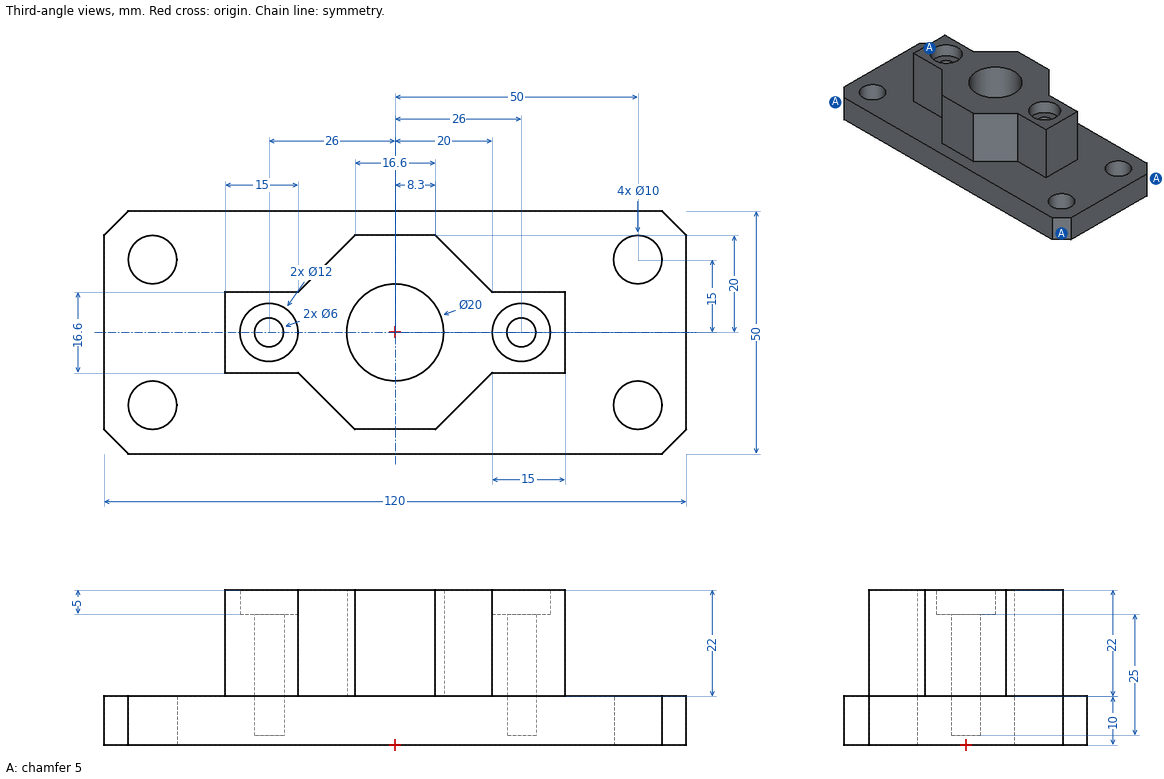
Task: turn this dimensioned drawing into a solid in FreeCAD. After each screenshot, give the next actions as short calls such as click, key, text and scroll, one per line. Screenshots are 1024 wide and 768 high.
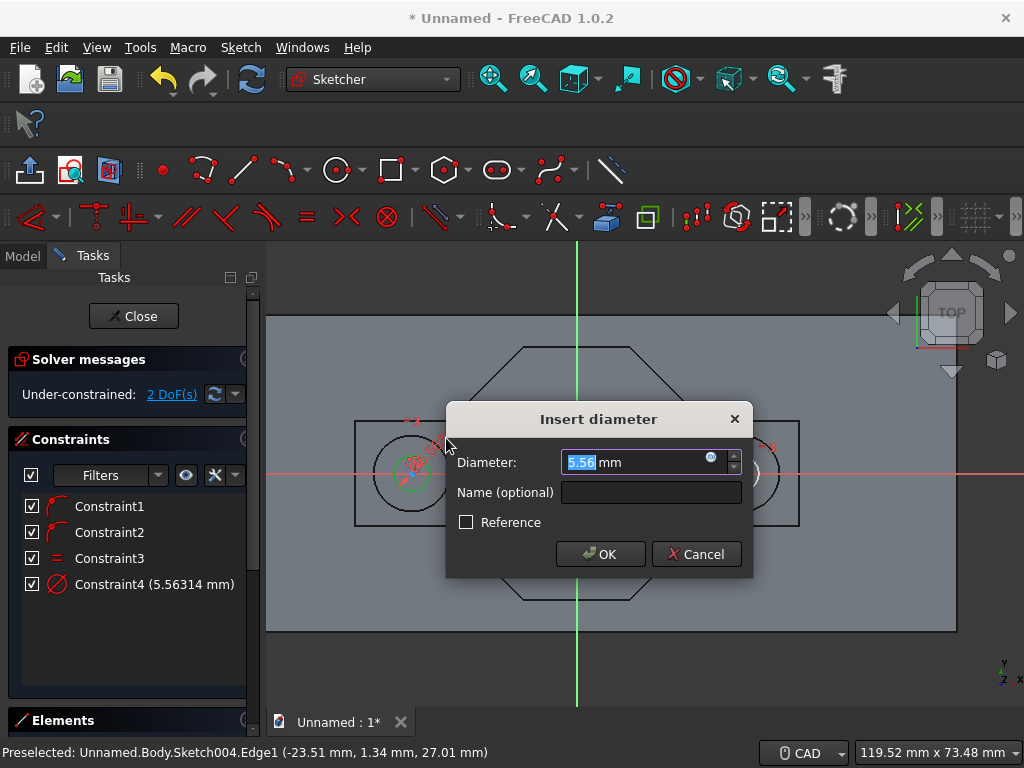
text(6)
key(Return)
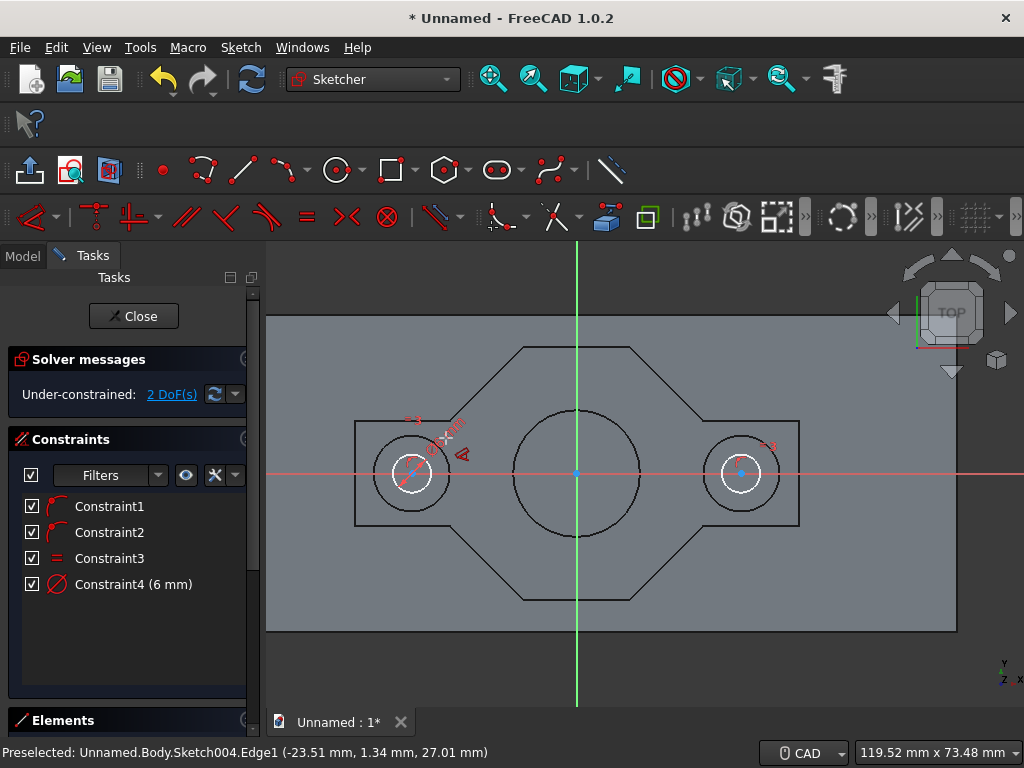
click(412, 474)
click(494, 508)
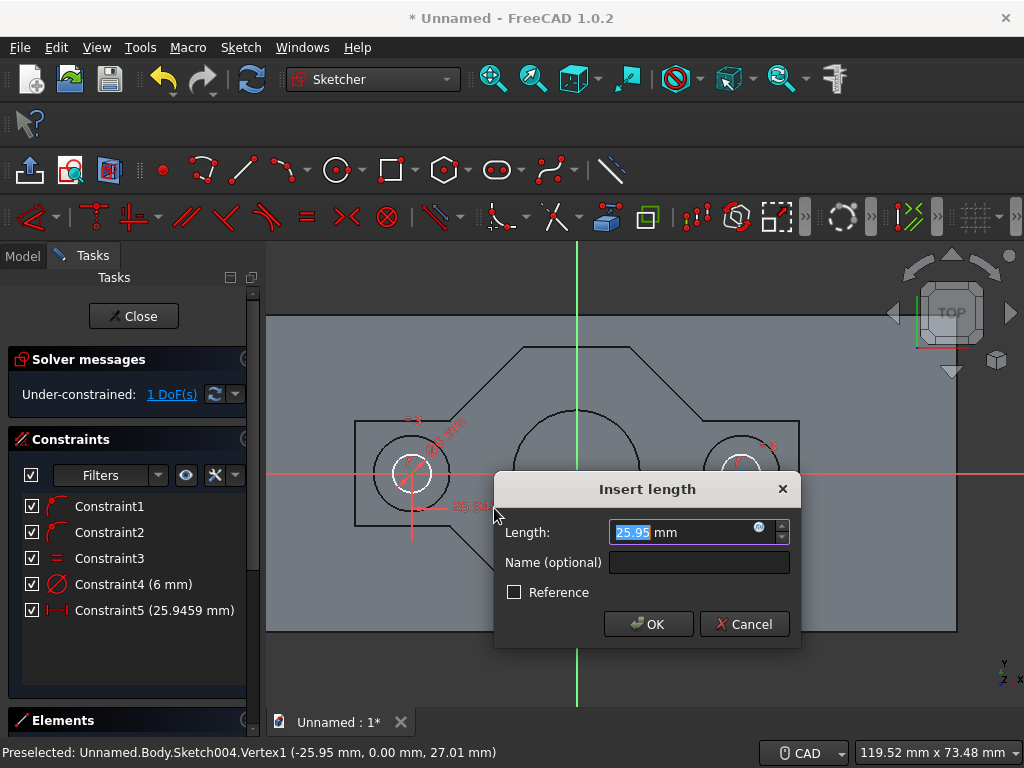
text(26)
key(Return)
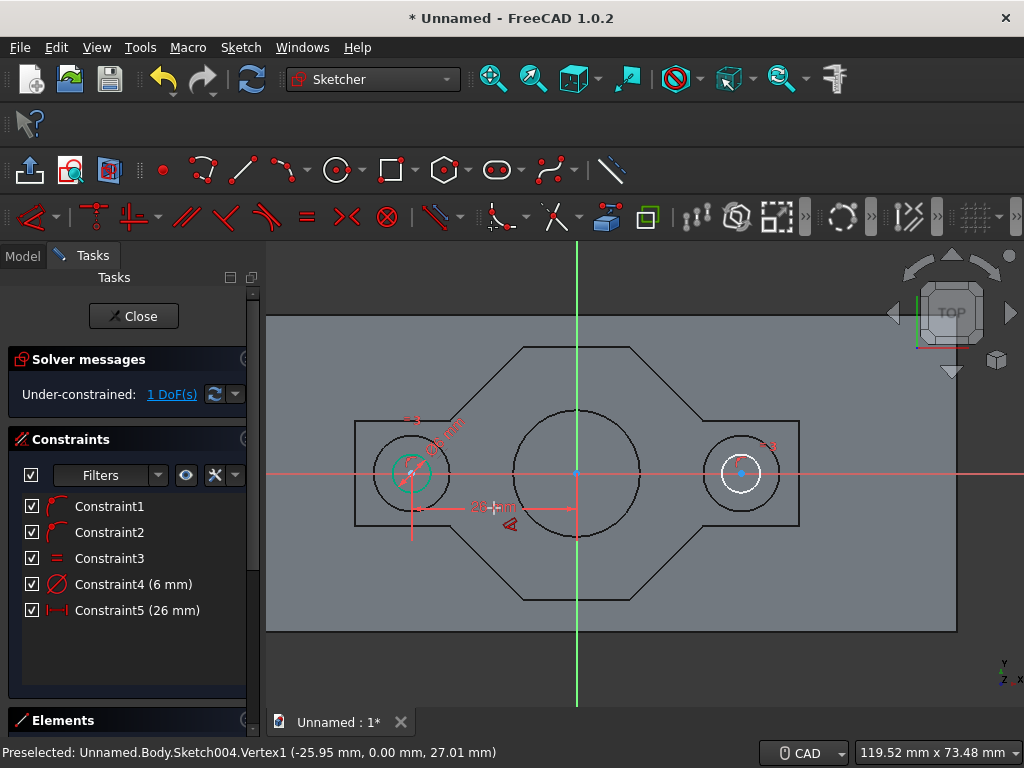
click(741, 474)
click(659, 508)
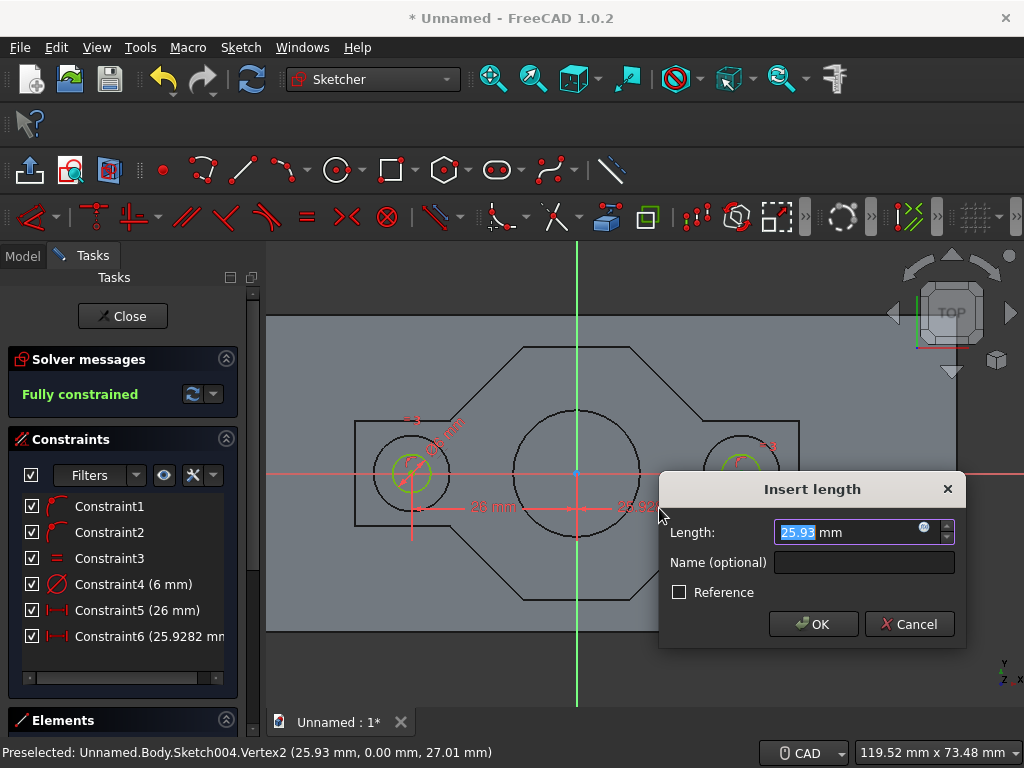
text(26)
key(Return)
key(Escape)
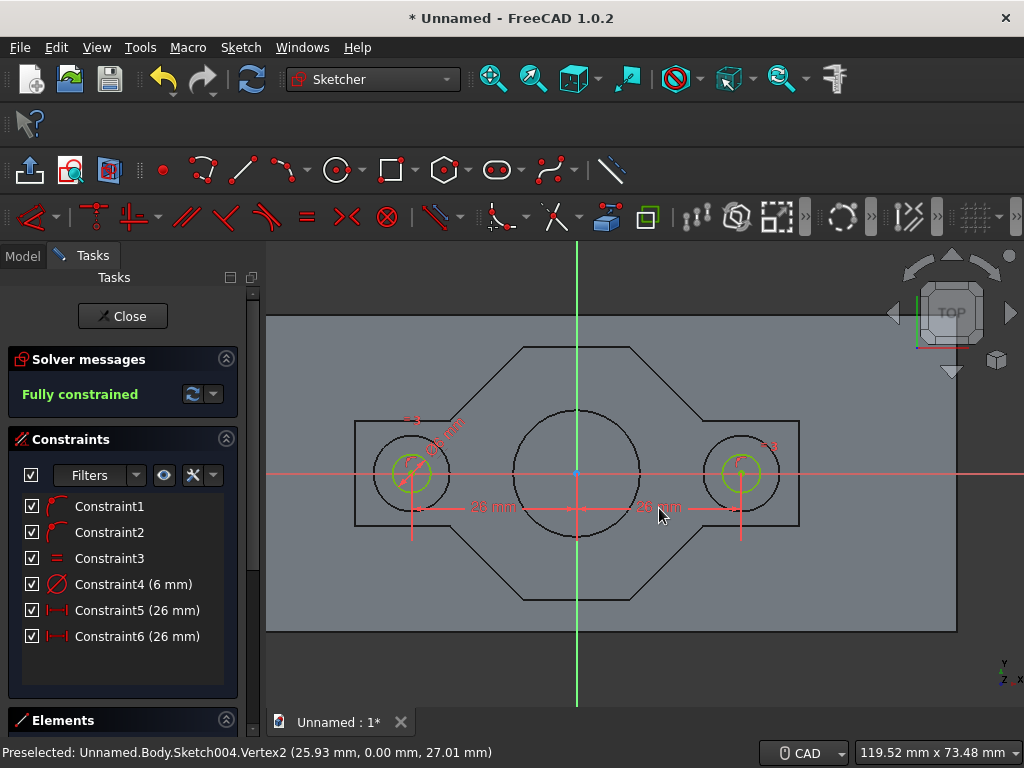
click(123, 316)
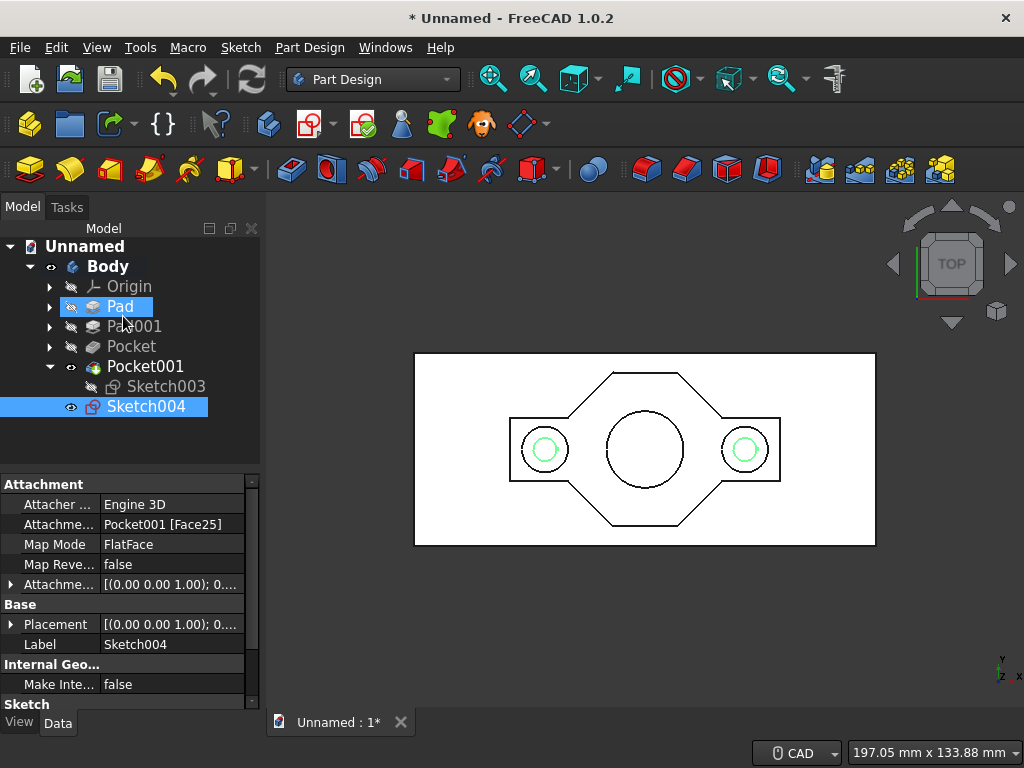
click(292, 170)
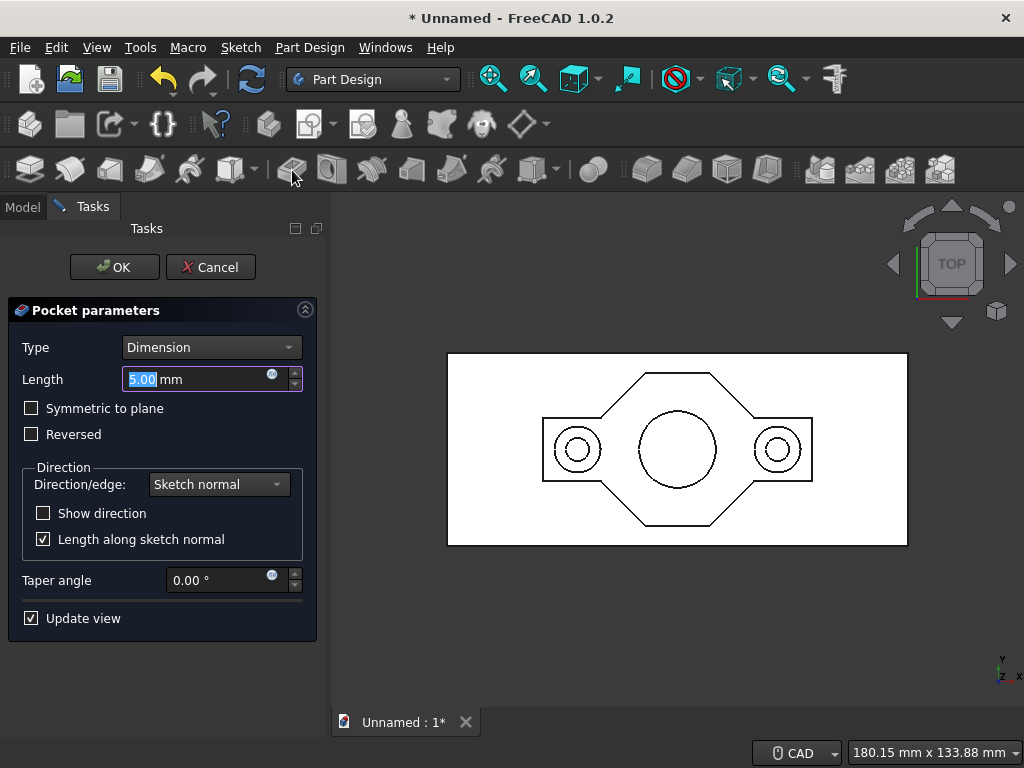
text(25)
key(Tab)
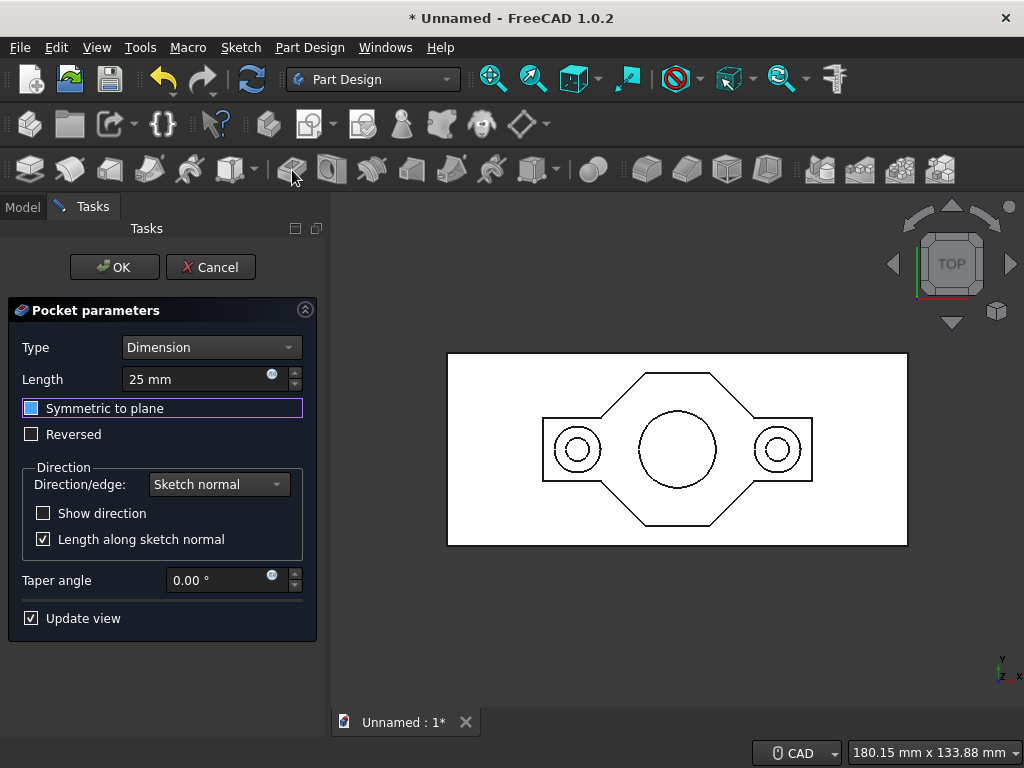
click(115, 267)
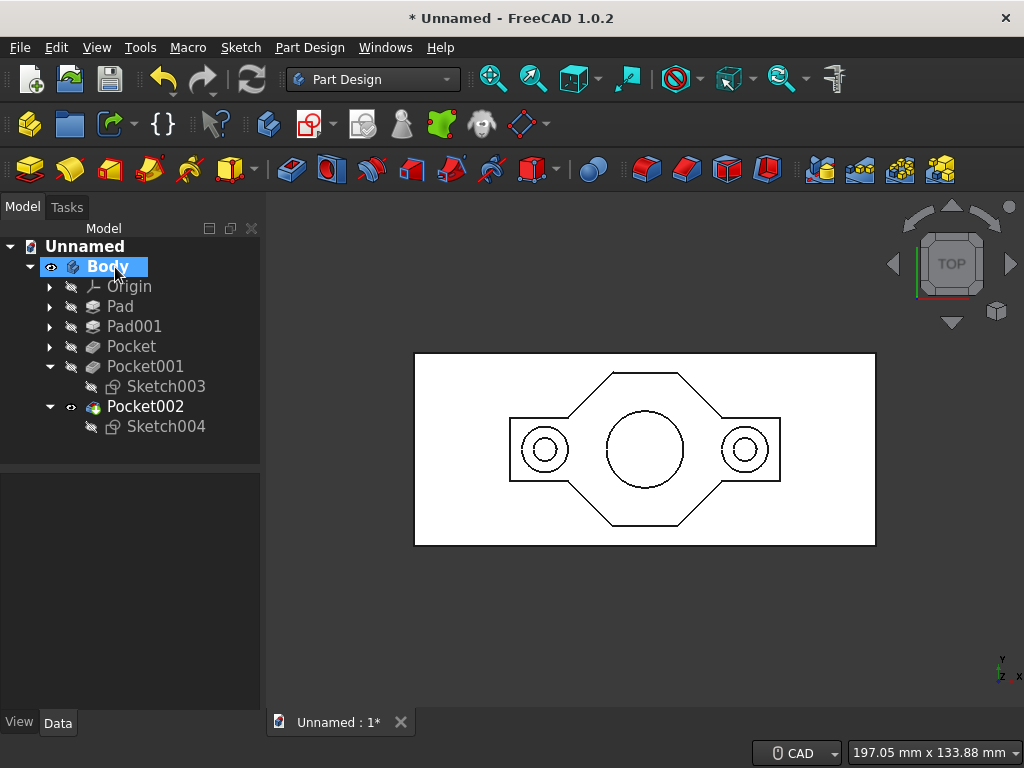
click(843, 394)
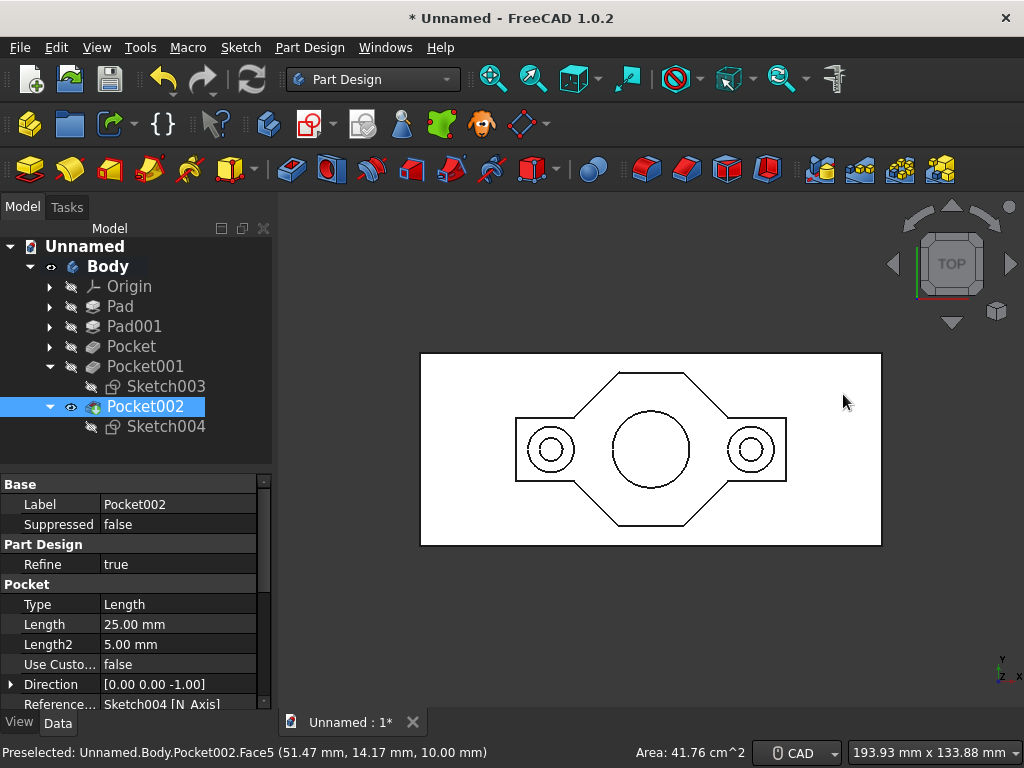
click(310, 124)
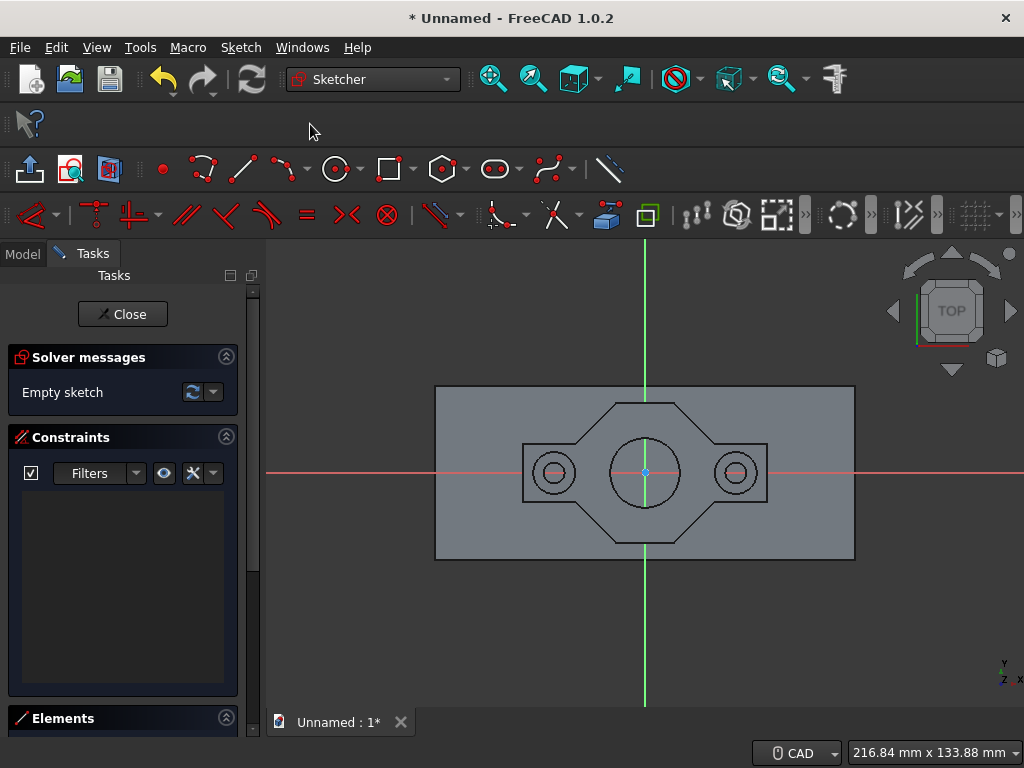
click(110, 170)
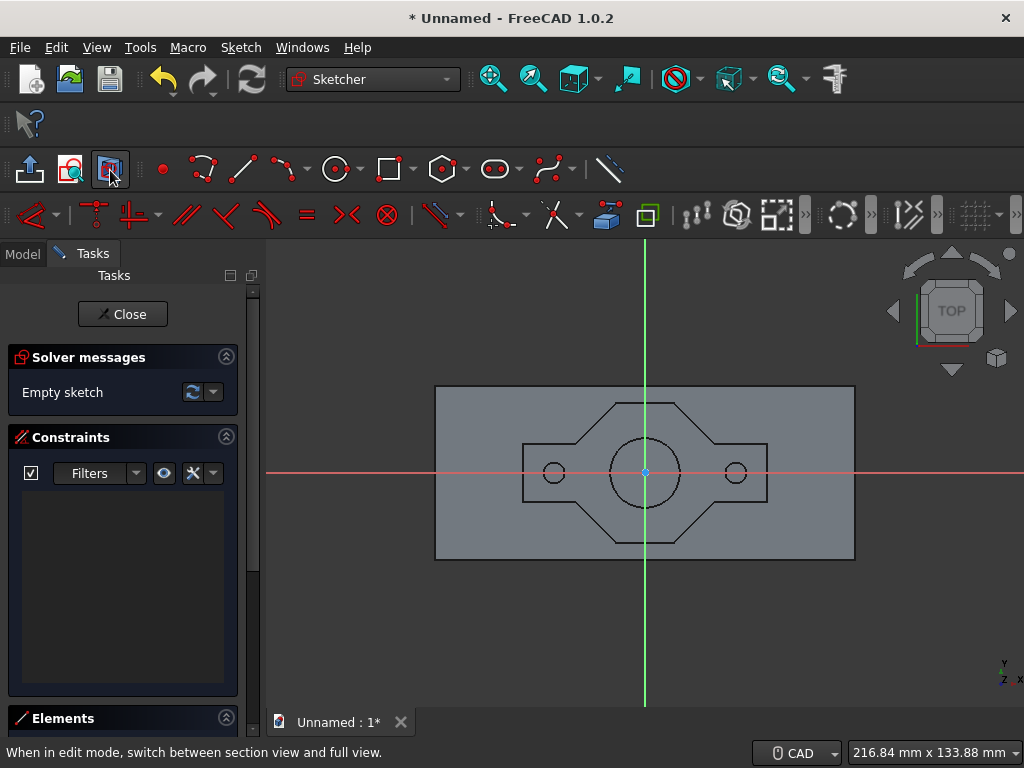
scroll(294, 473, down, 1)